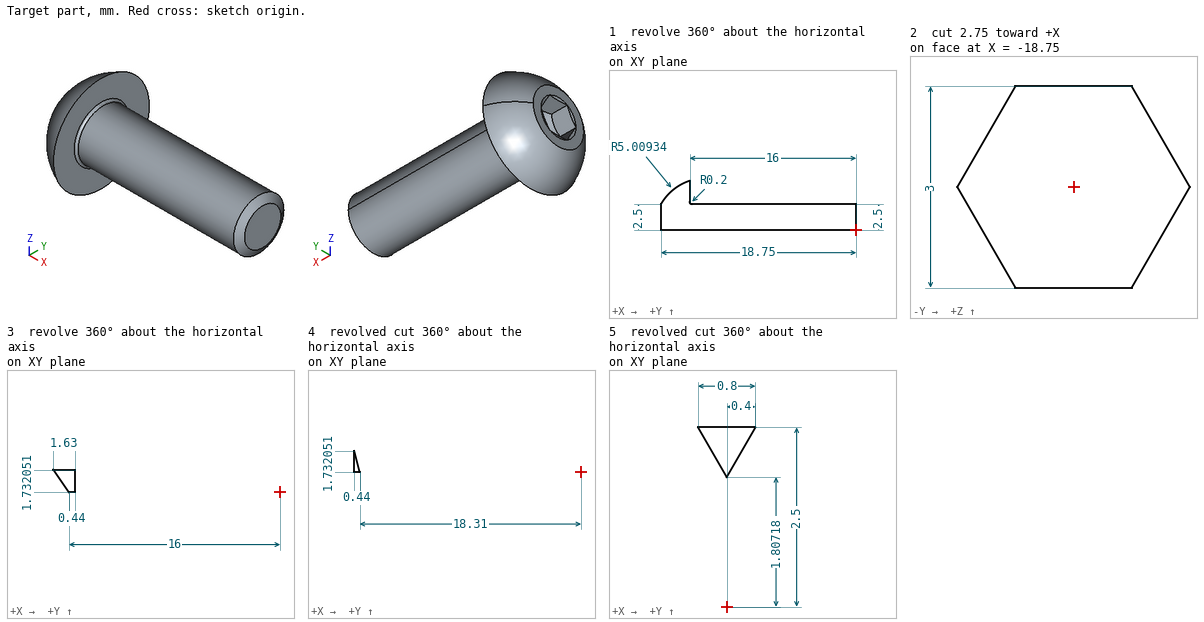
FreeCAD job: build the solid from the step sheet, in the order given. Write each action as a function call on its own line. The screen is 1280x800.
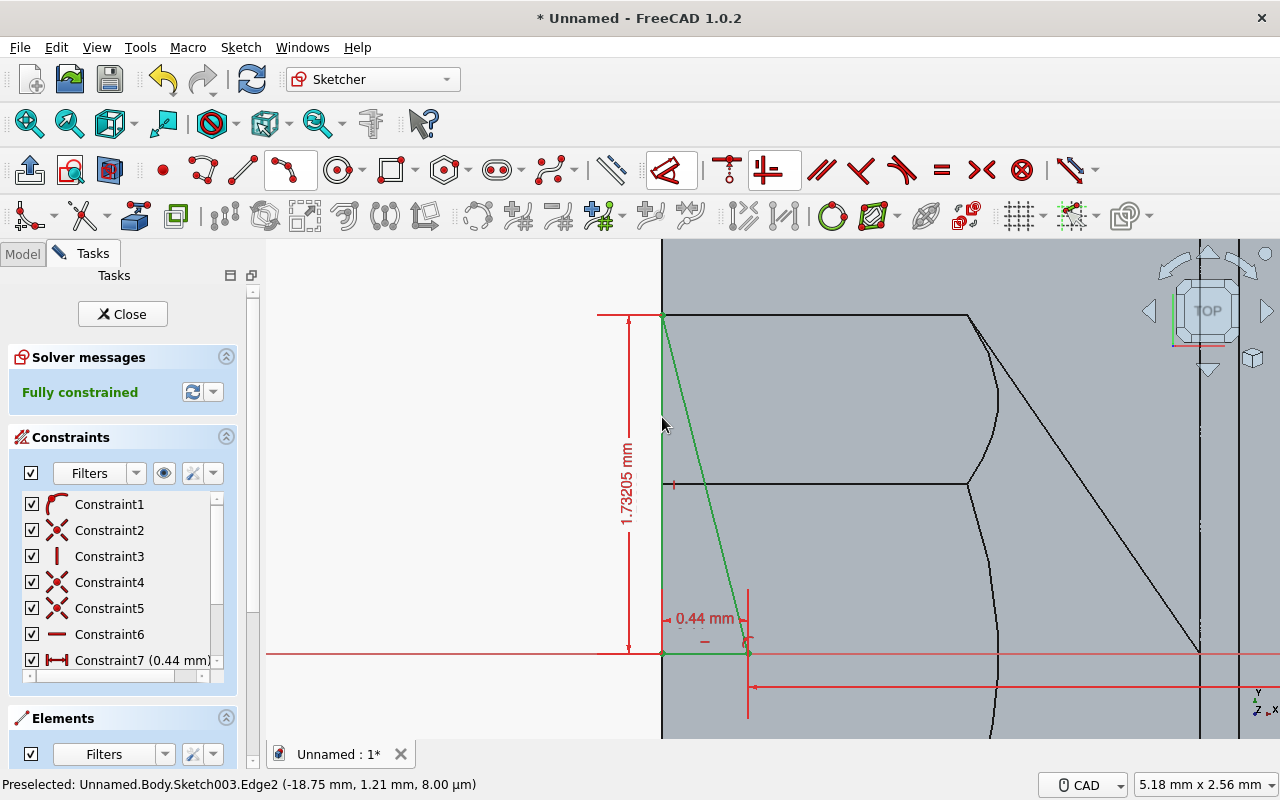
click(123, 314)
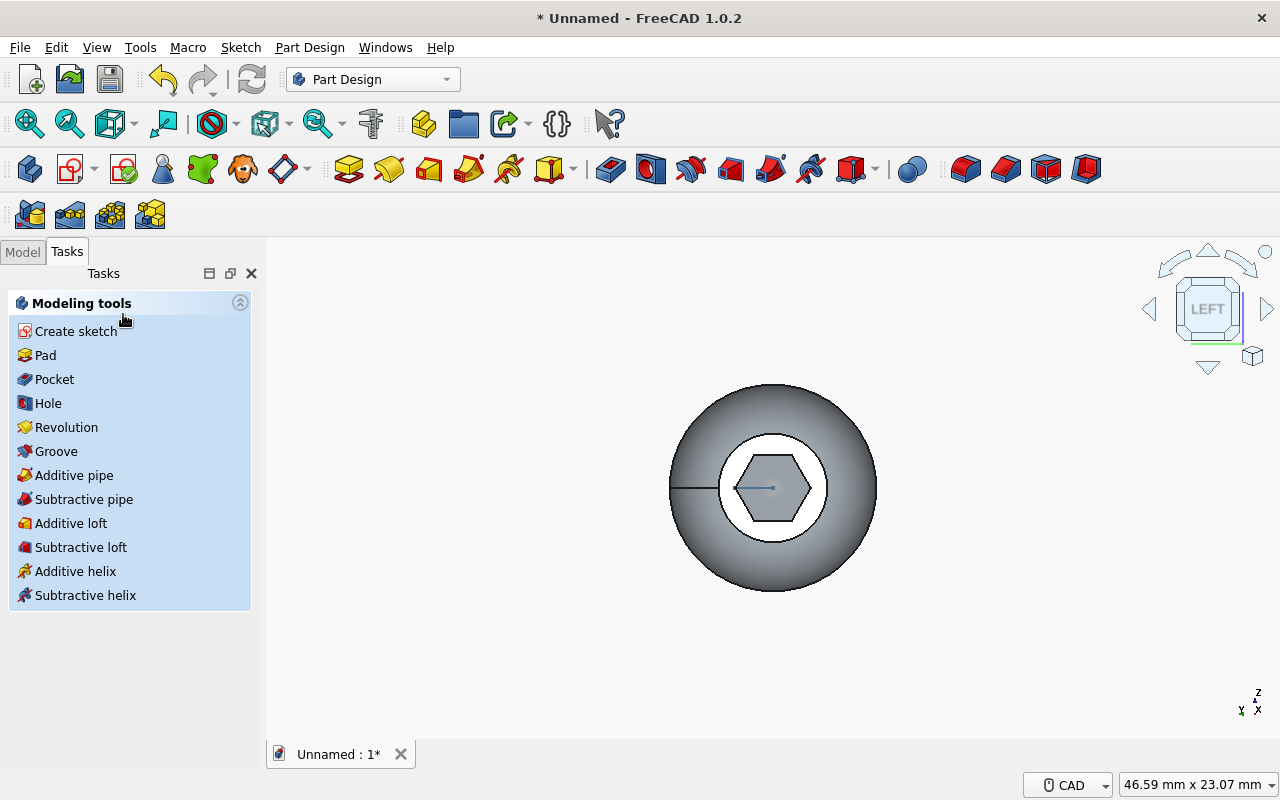
click(692, 170)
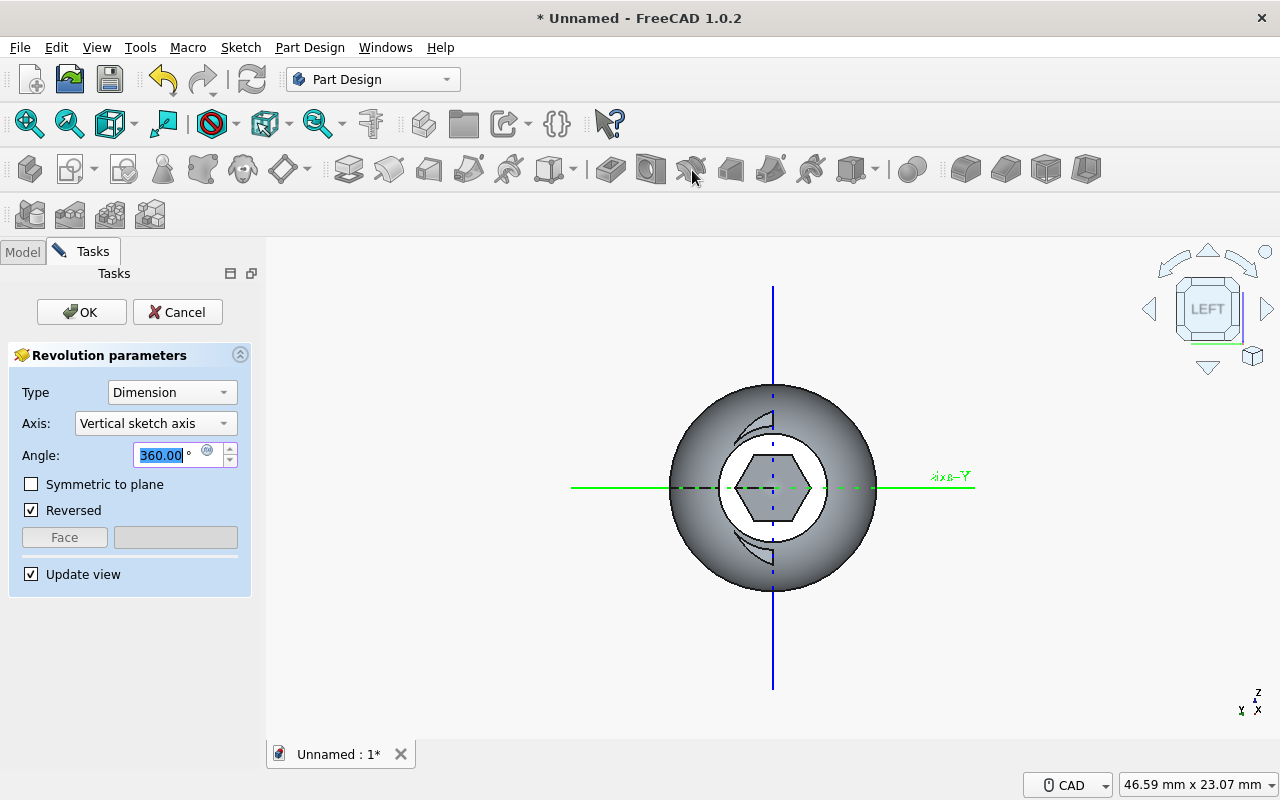
click(156, 424)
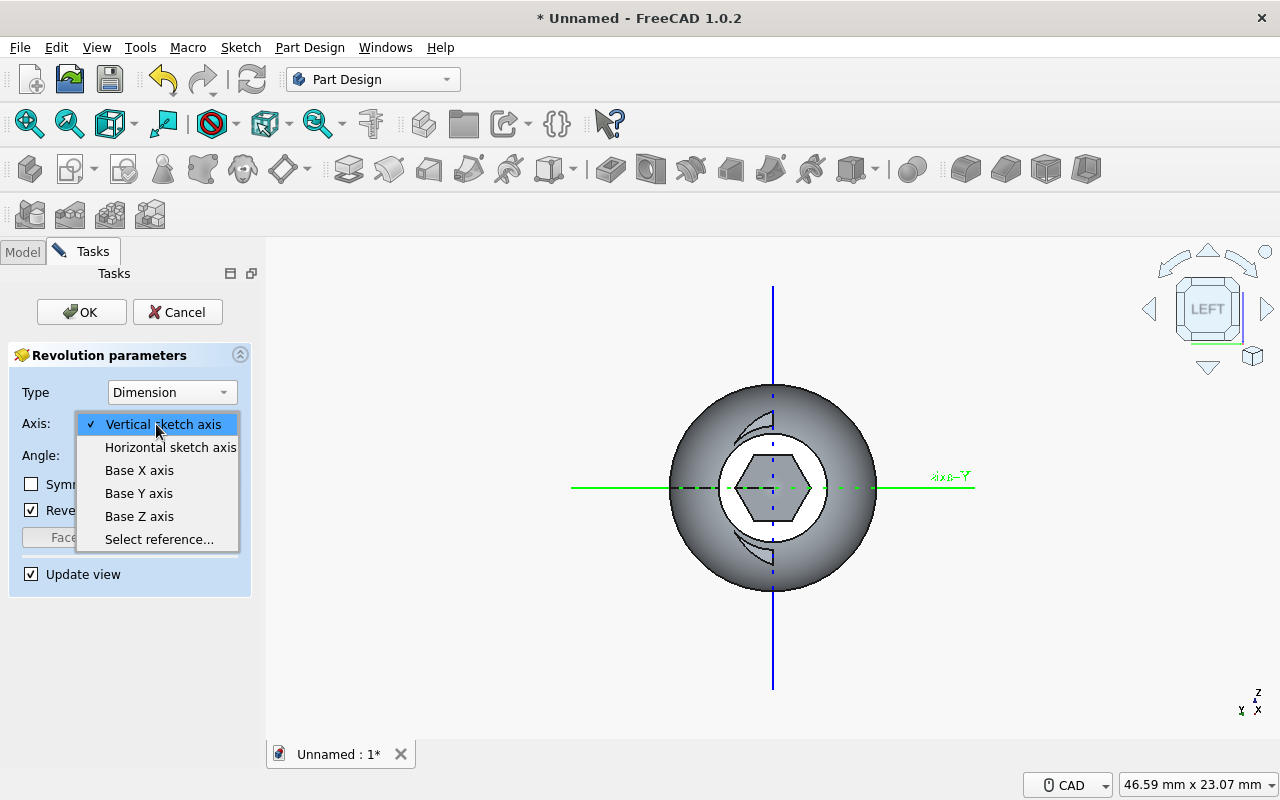
click(156, 448)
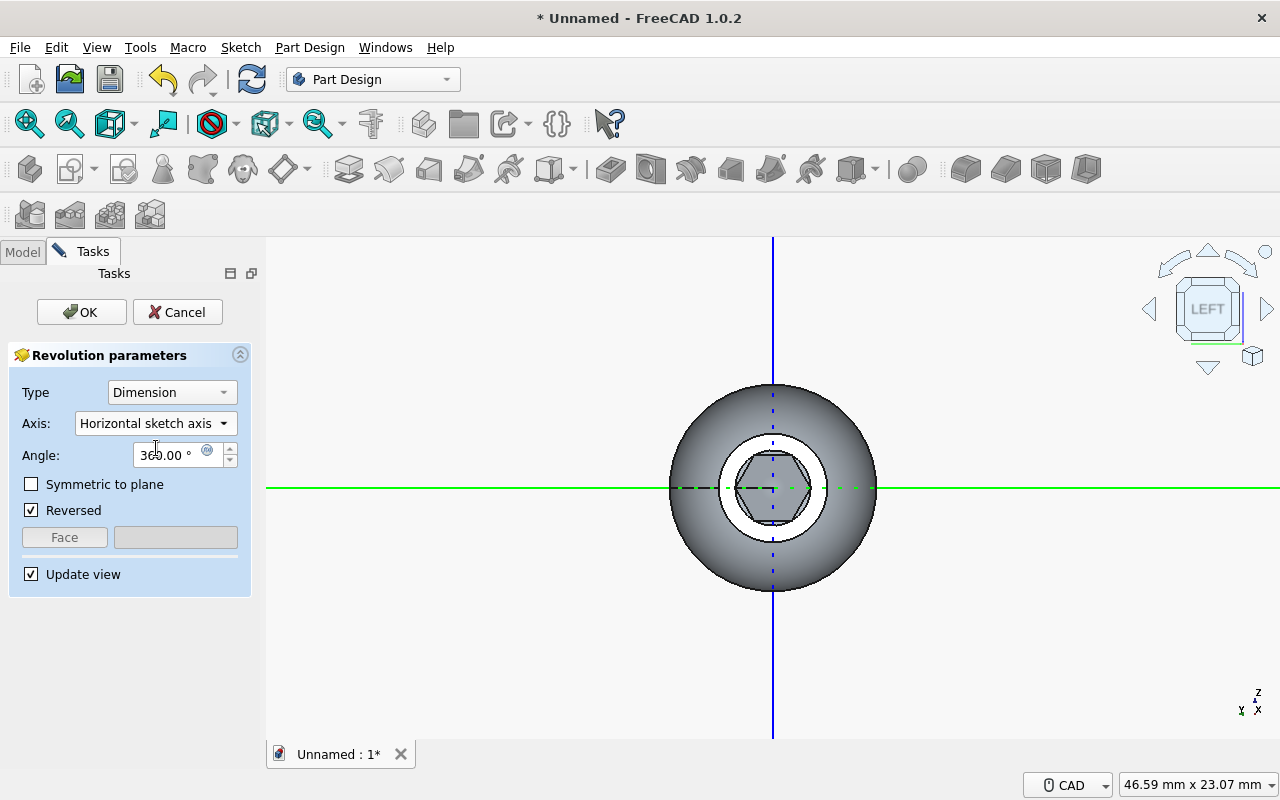
click(82, 312)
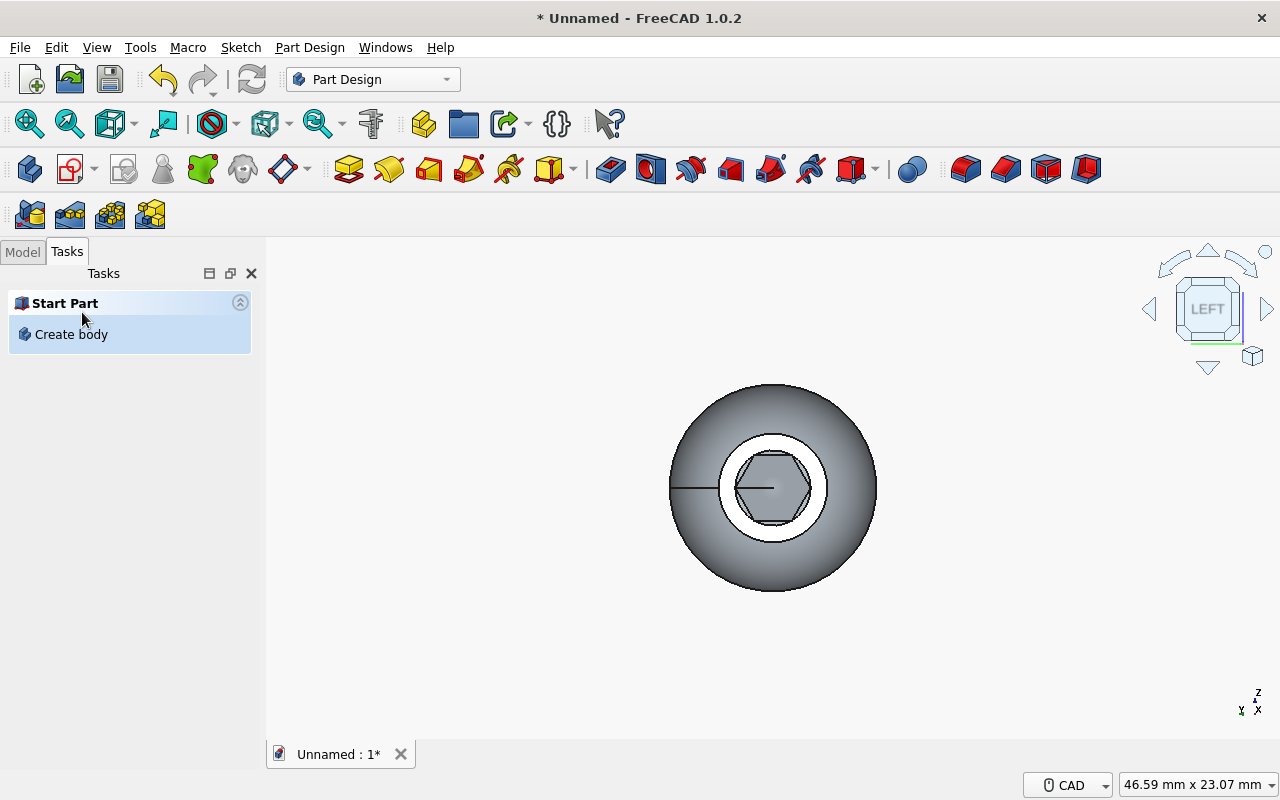
click(30, 124)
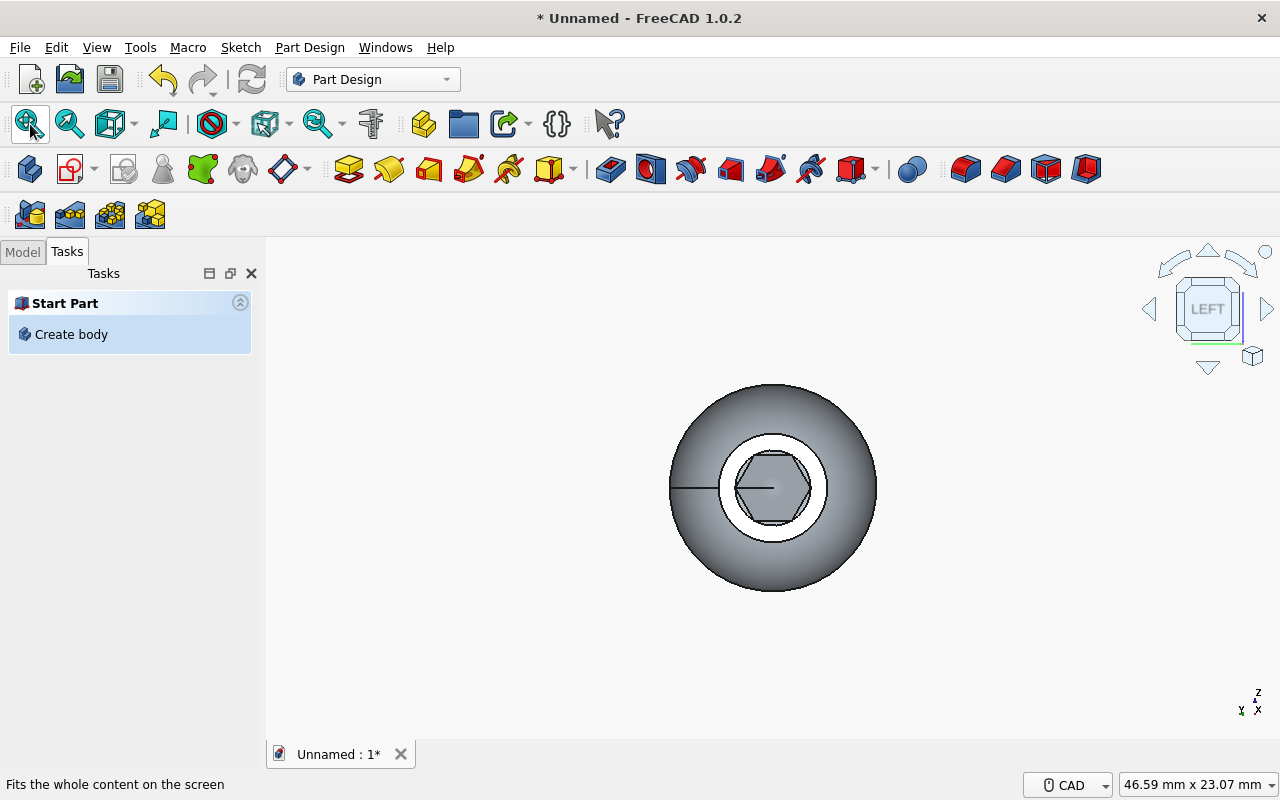
click(70, 170)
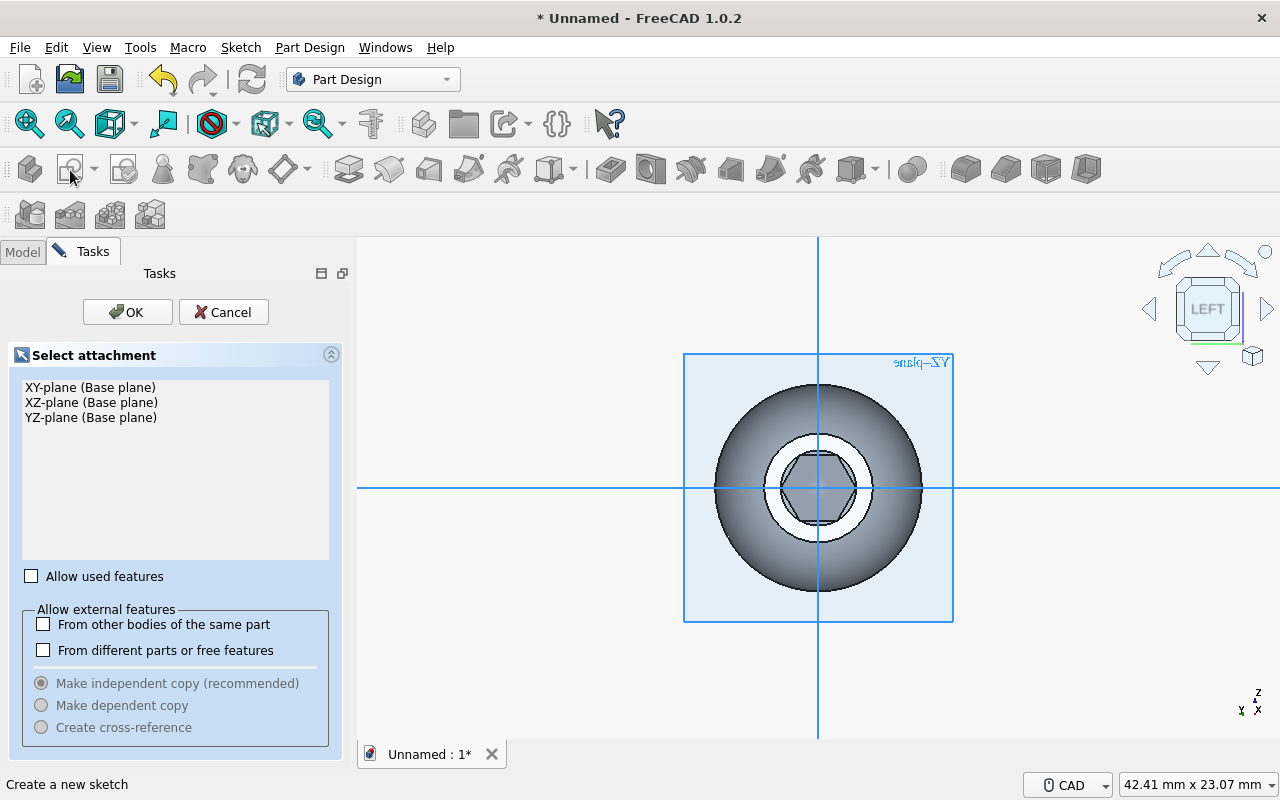
click(82, 388)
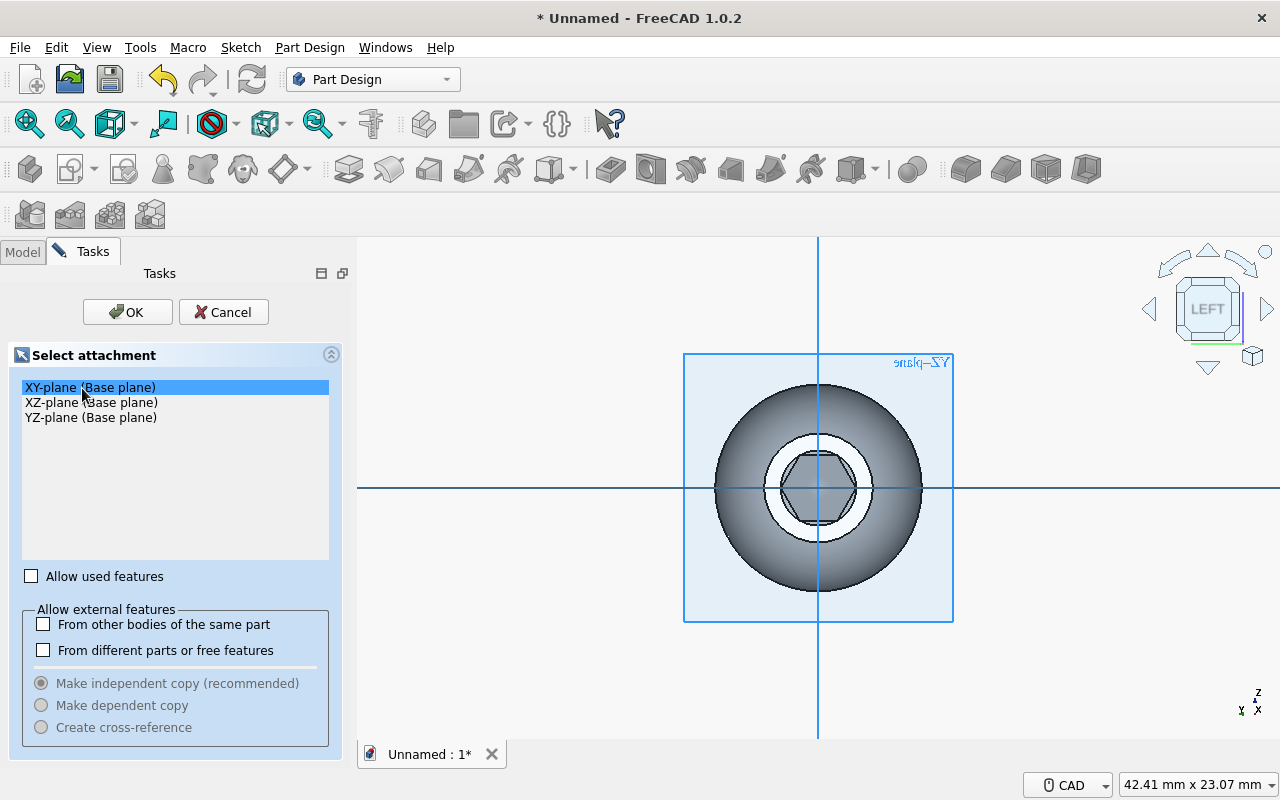
click(128, 312)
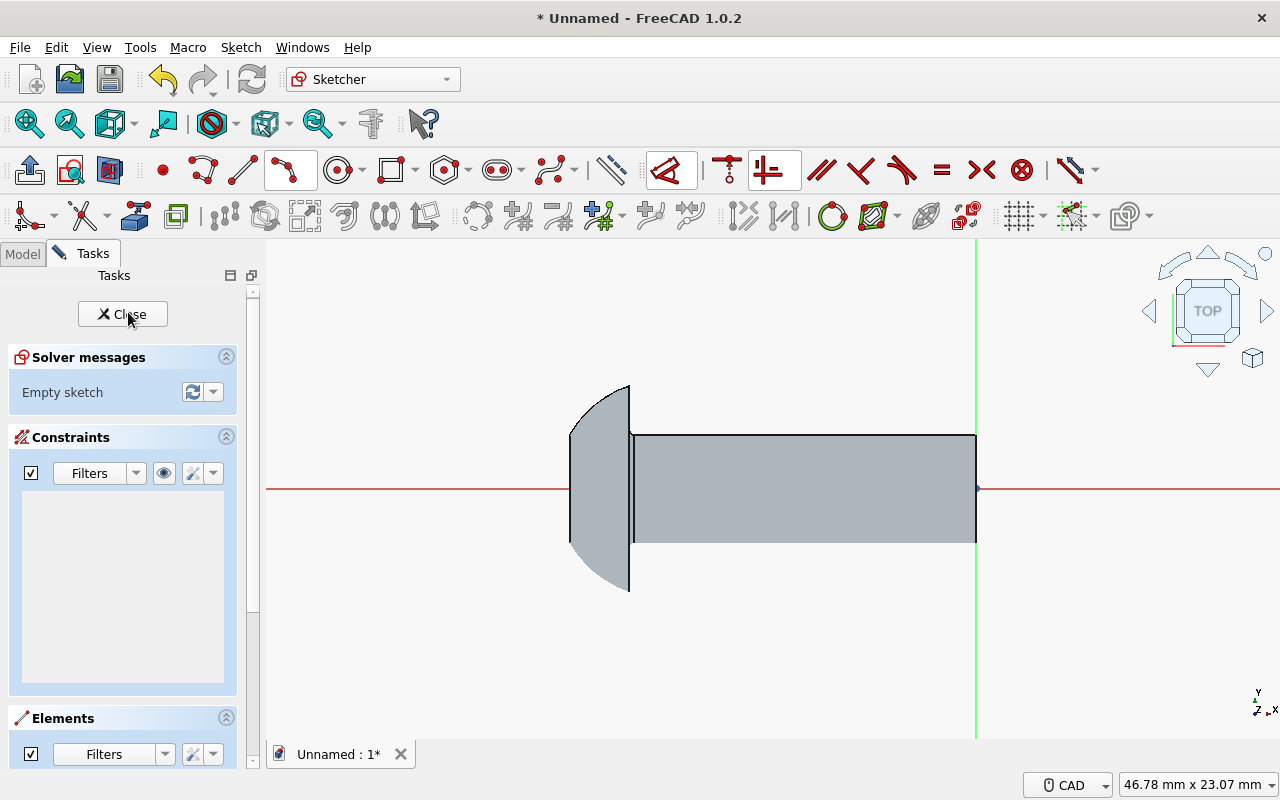
click(110, 170)